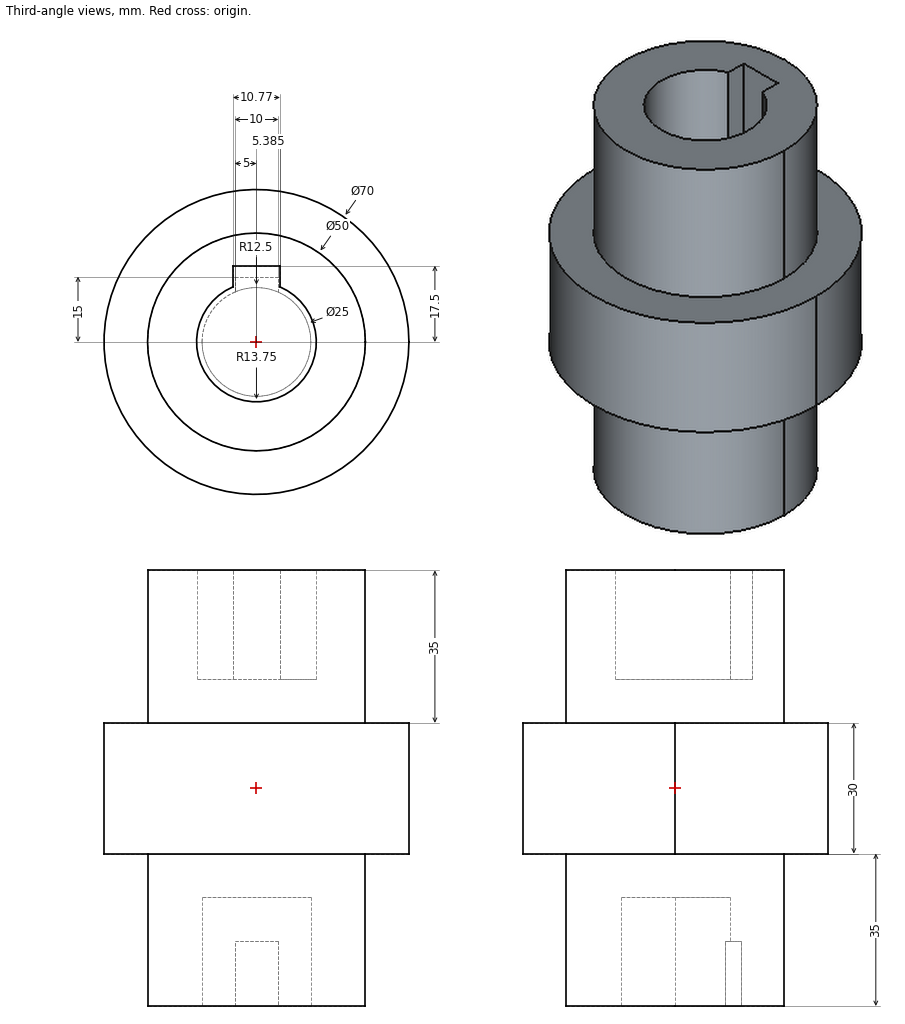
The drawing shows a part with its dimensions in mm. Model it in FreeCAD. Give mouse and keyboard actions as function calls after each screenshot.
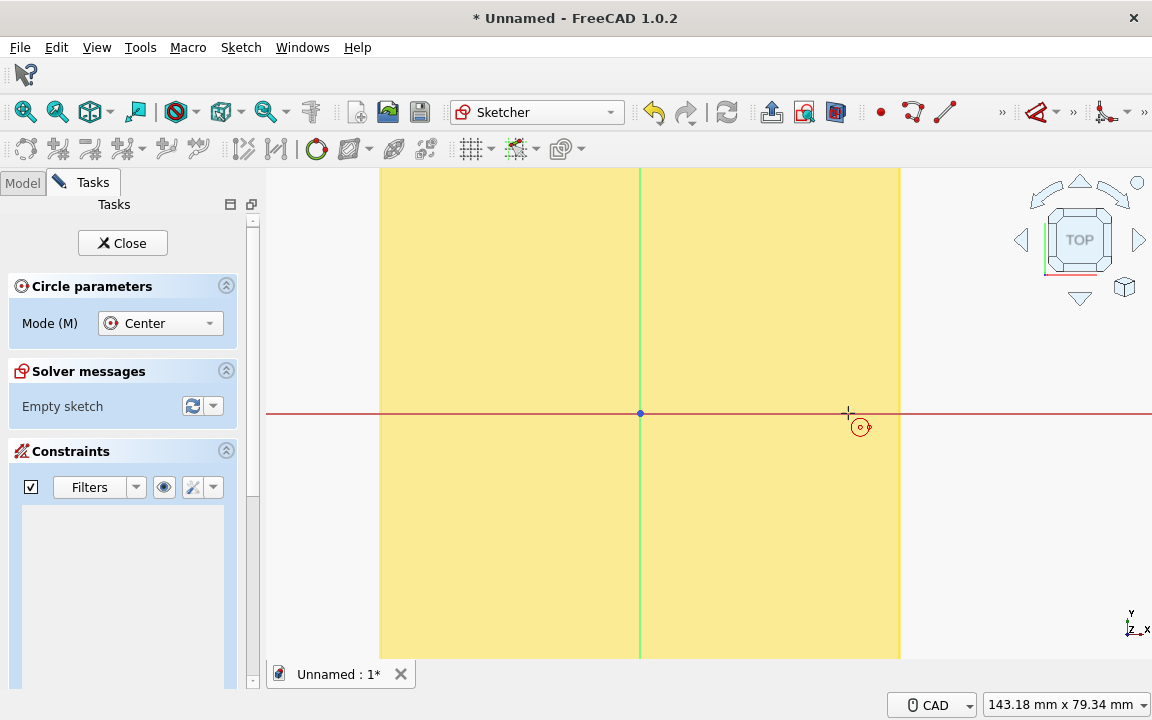
click(640, 414)
move(750, 304)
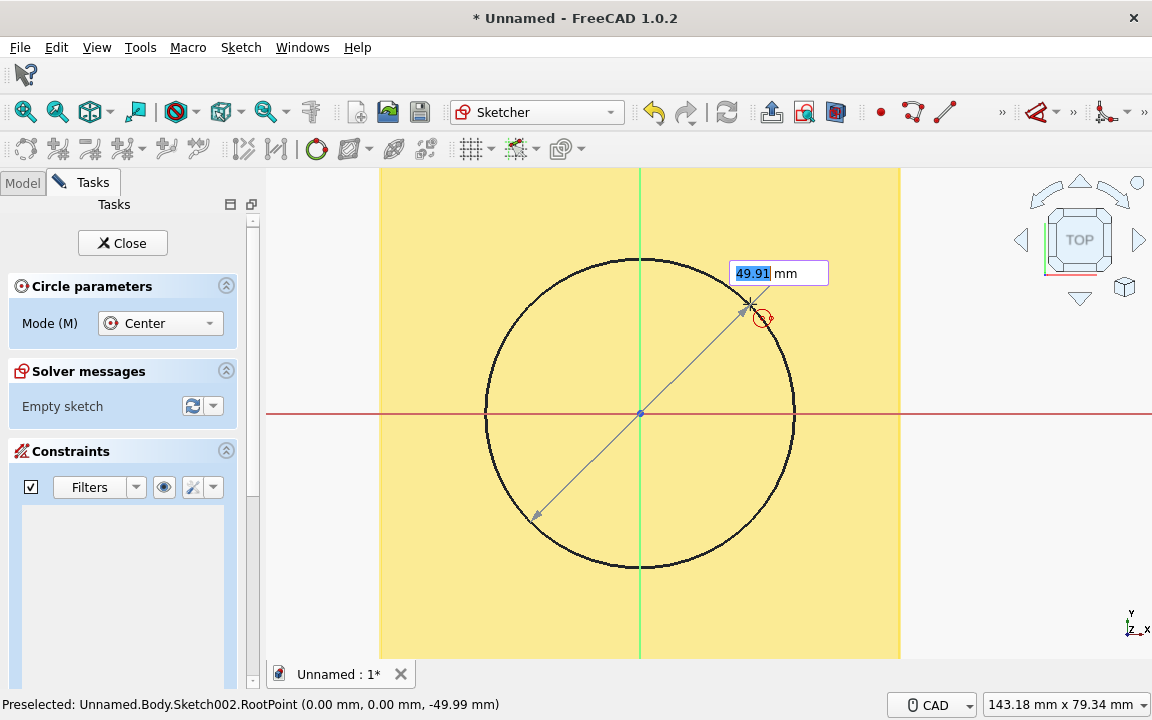
text(50)
key(Return)
key(Escape)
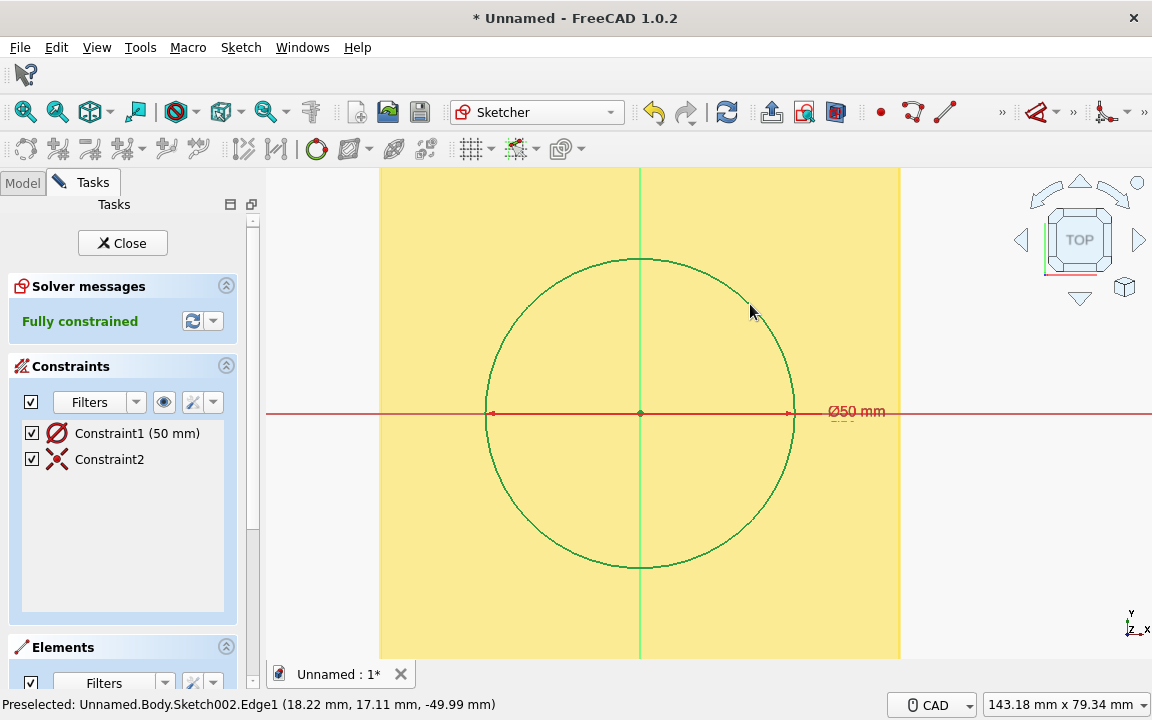
click(123, 243)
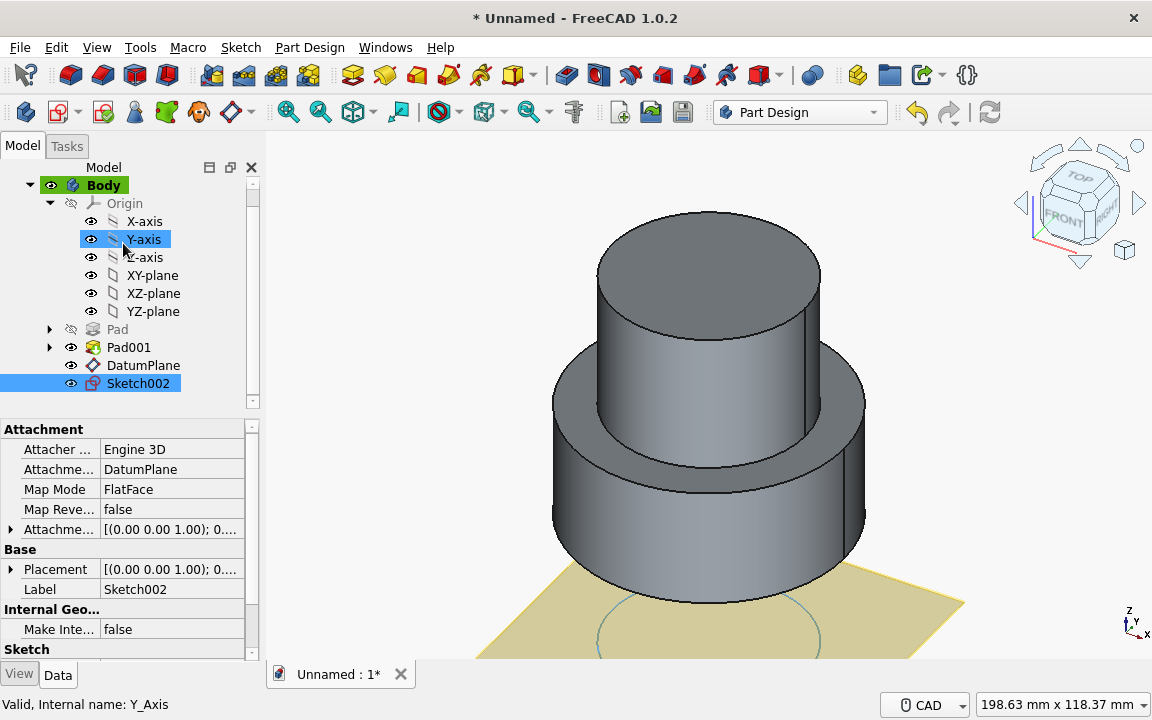
click(354, 76)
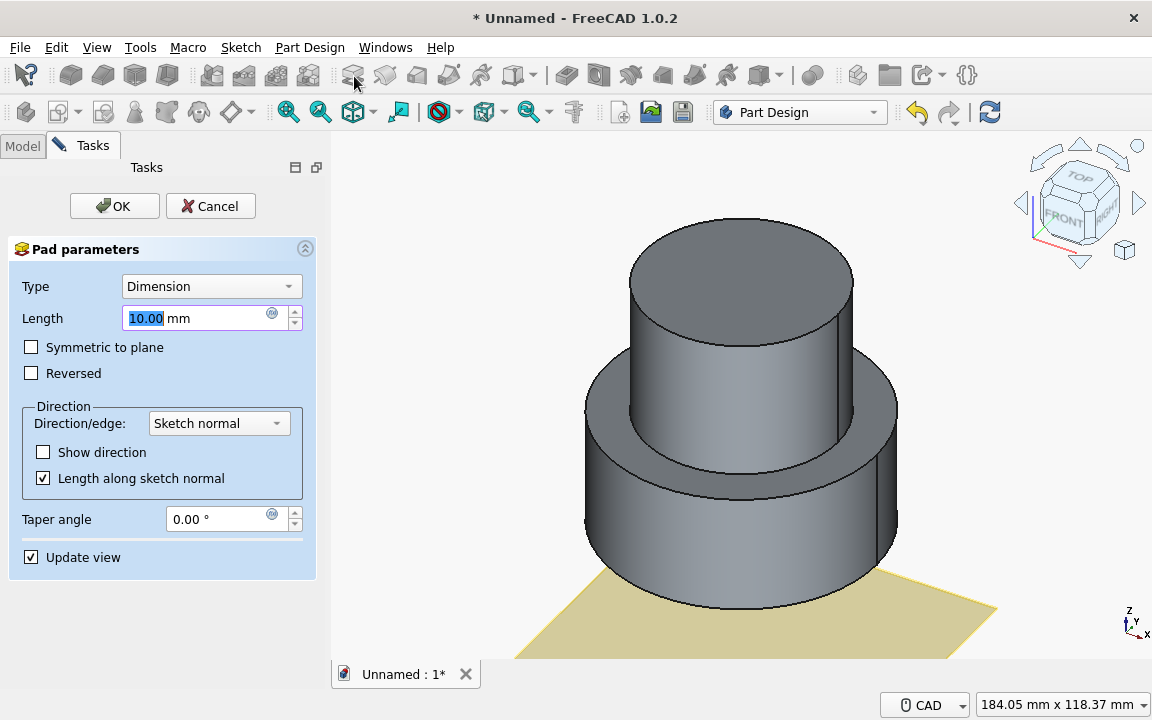
text(35)
key(Tab)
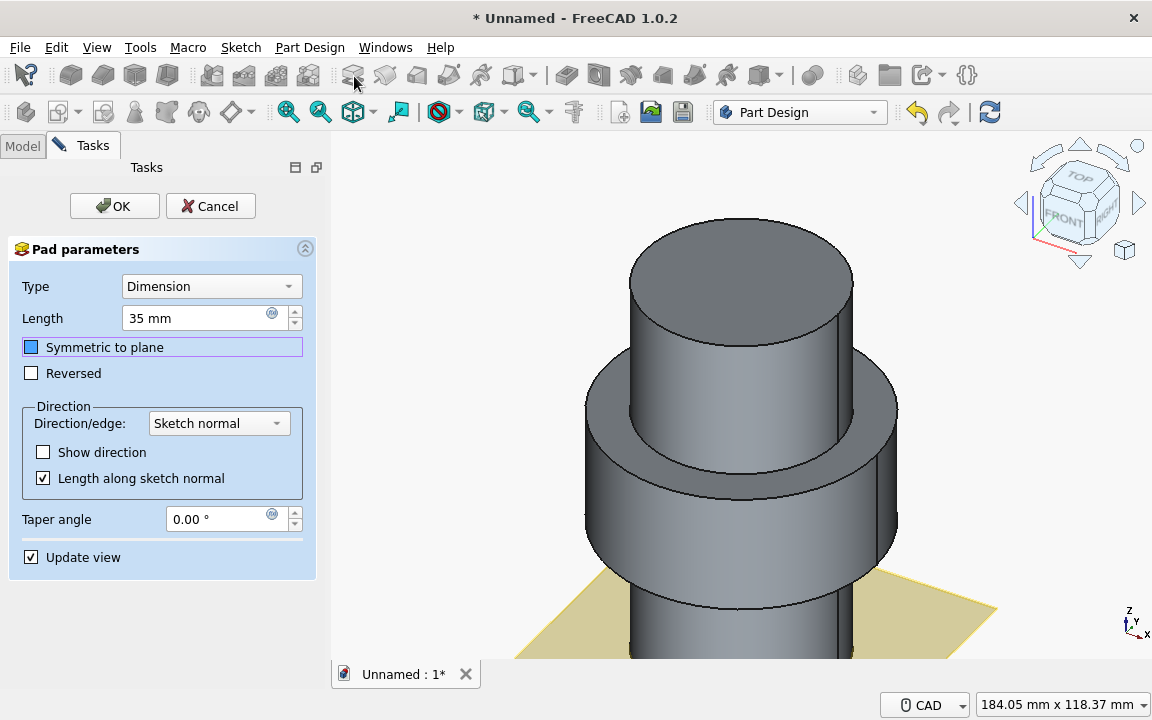
click(115, 206)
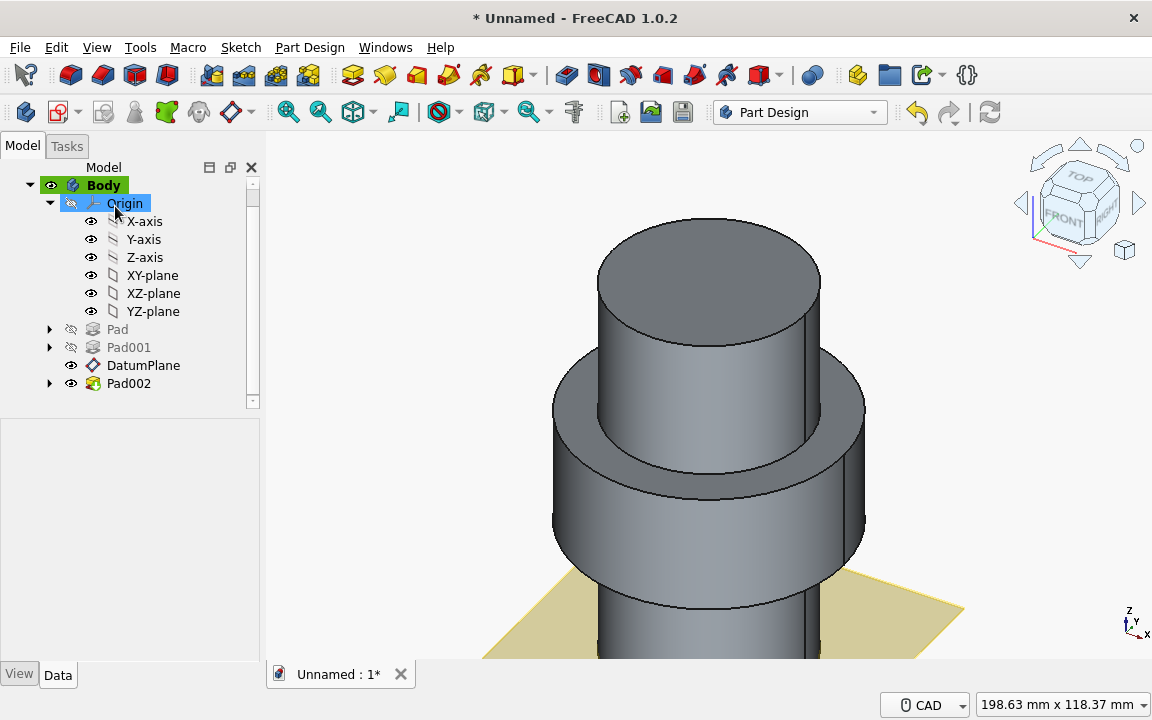
click(116, 365)
key(space)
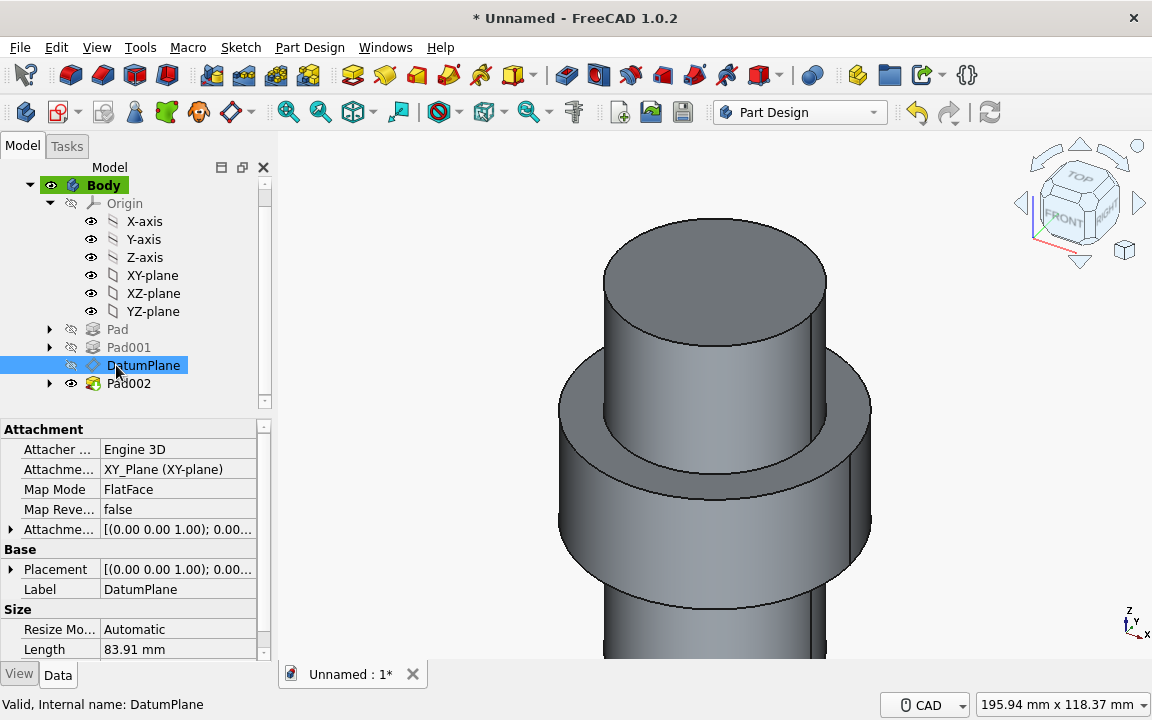
key(v)
key(f)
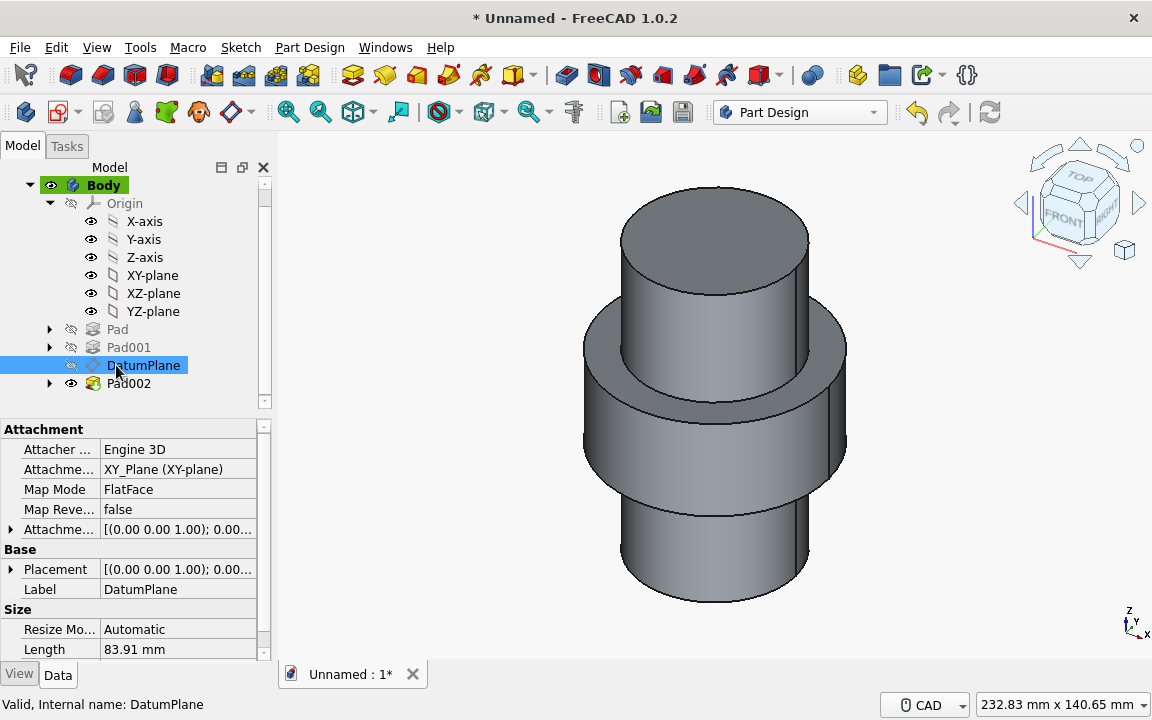
click(715, 240)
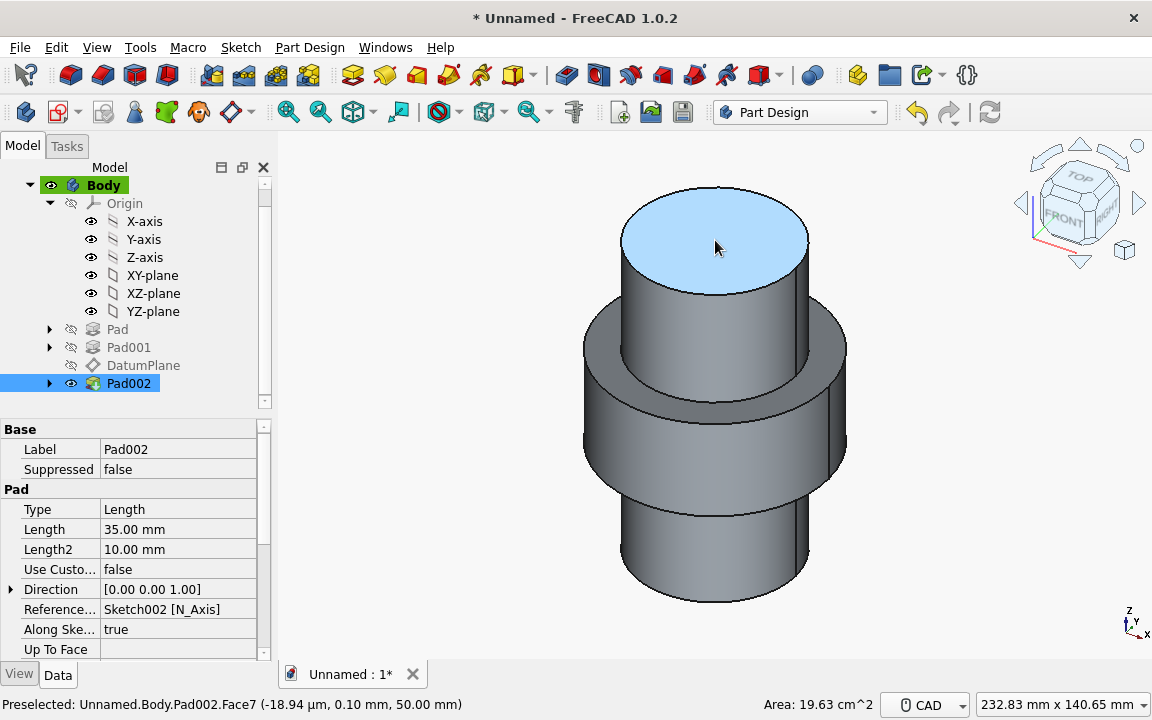
click(58, 112)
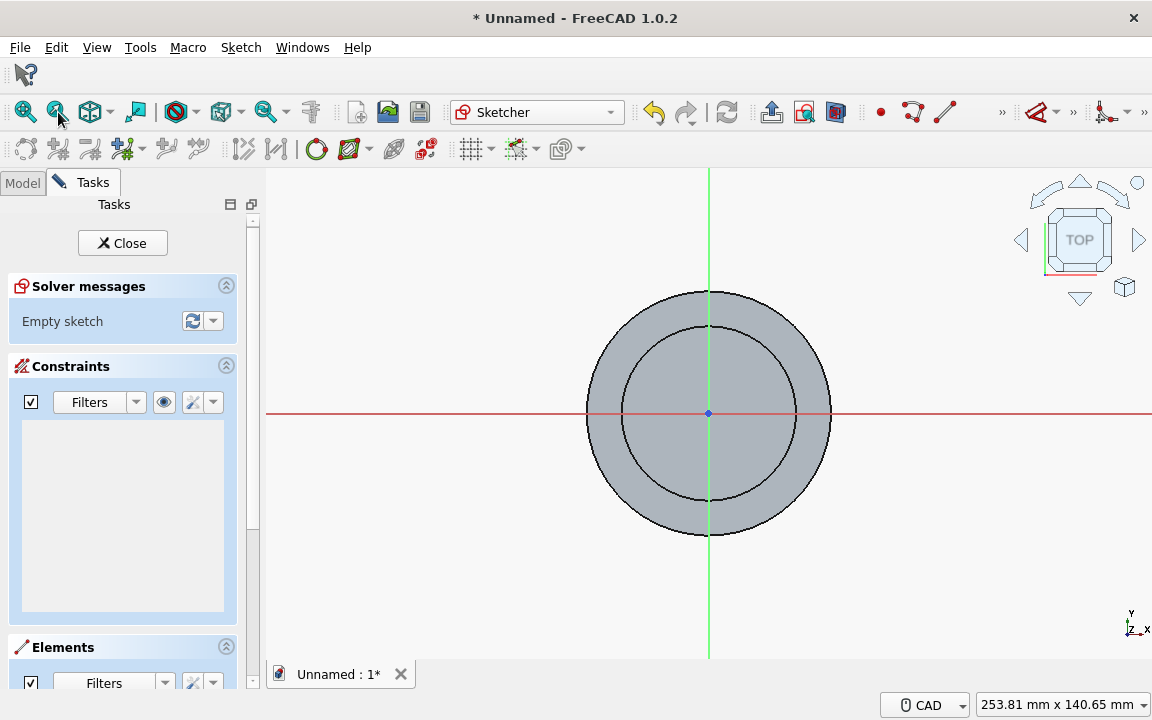
scroll(749, 403, up, 5)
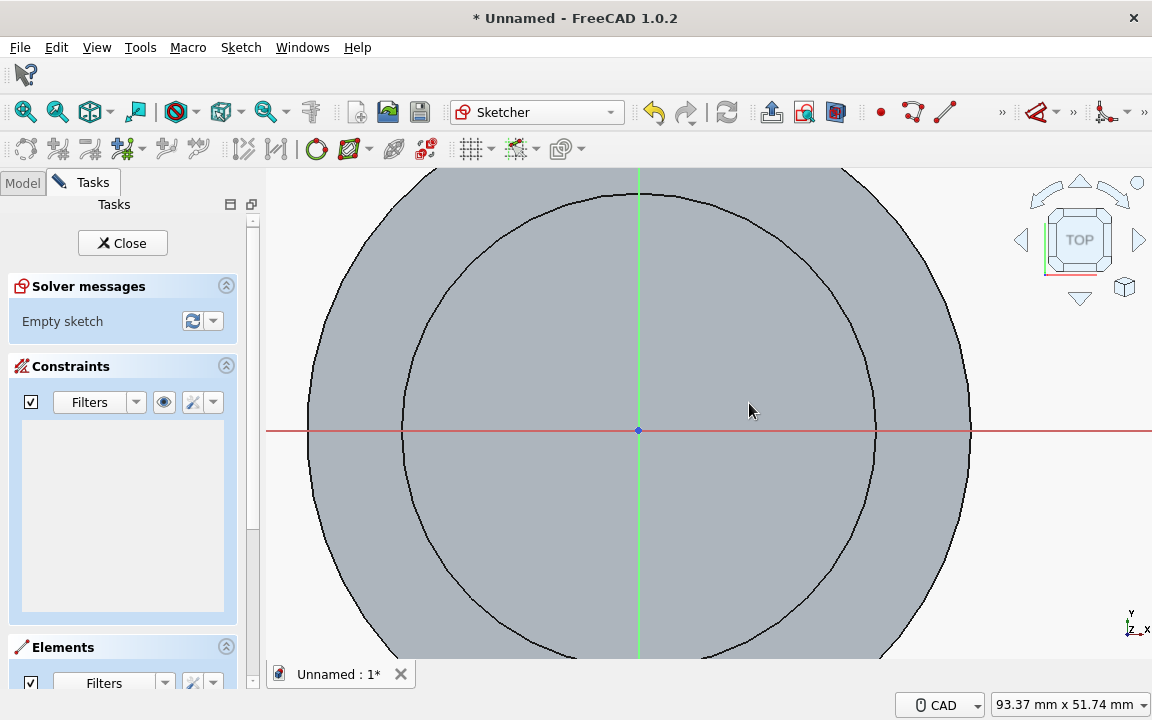
key(g)
key(m)